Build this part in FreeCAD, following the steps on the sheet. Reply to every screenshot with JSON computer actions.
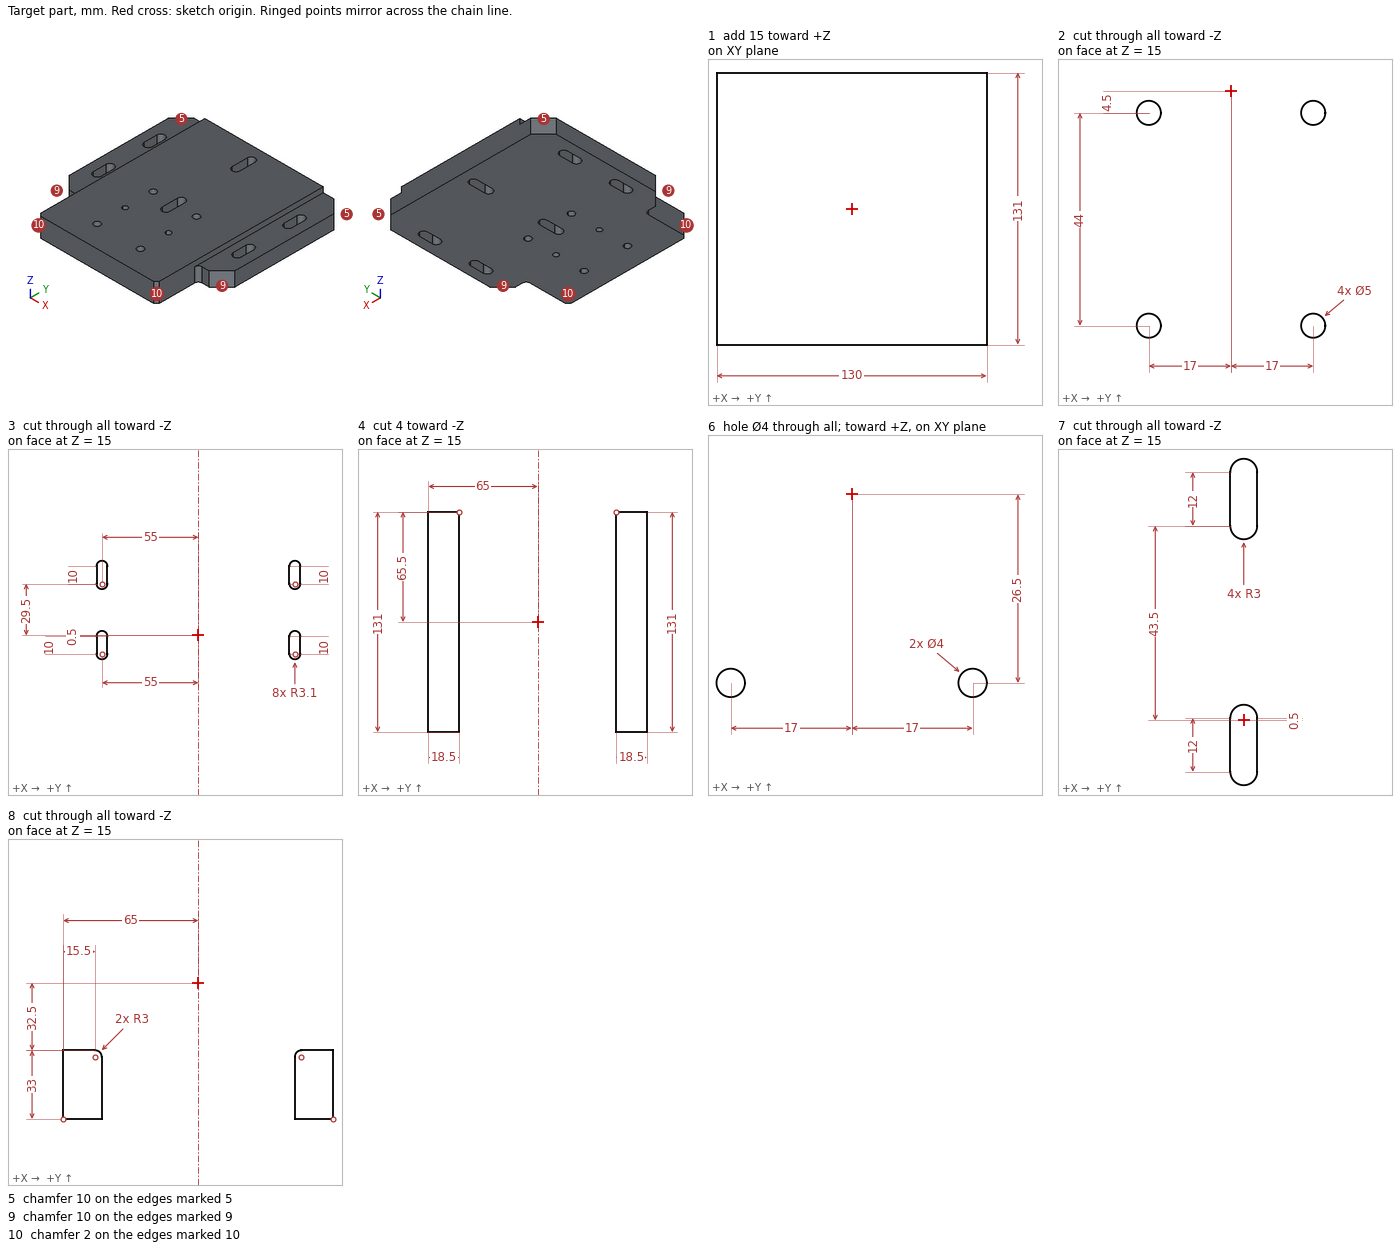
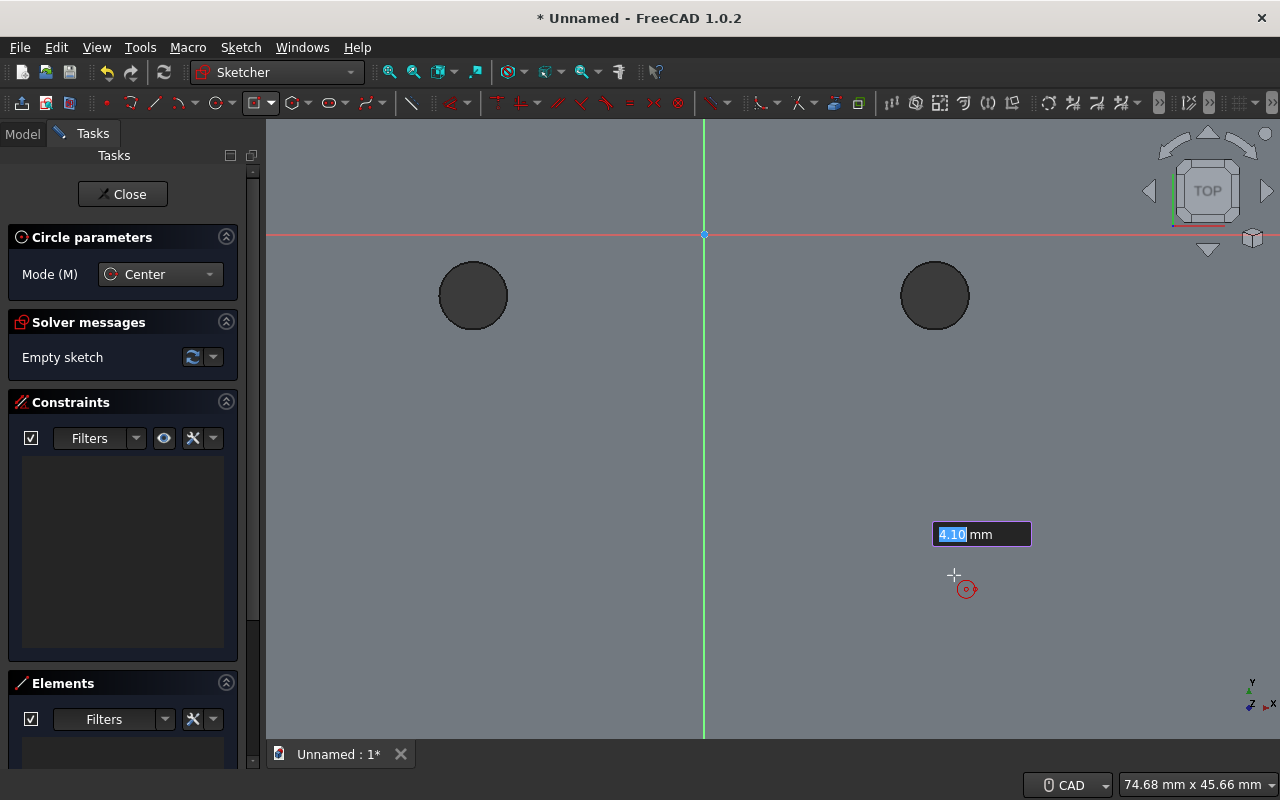
{"action": "type", "text": "4"}
{"action": "key", "text": "Return"}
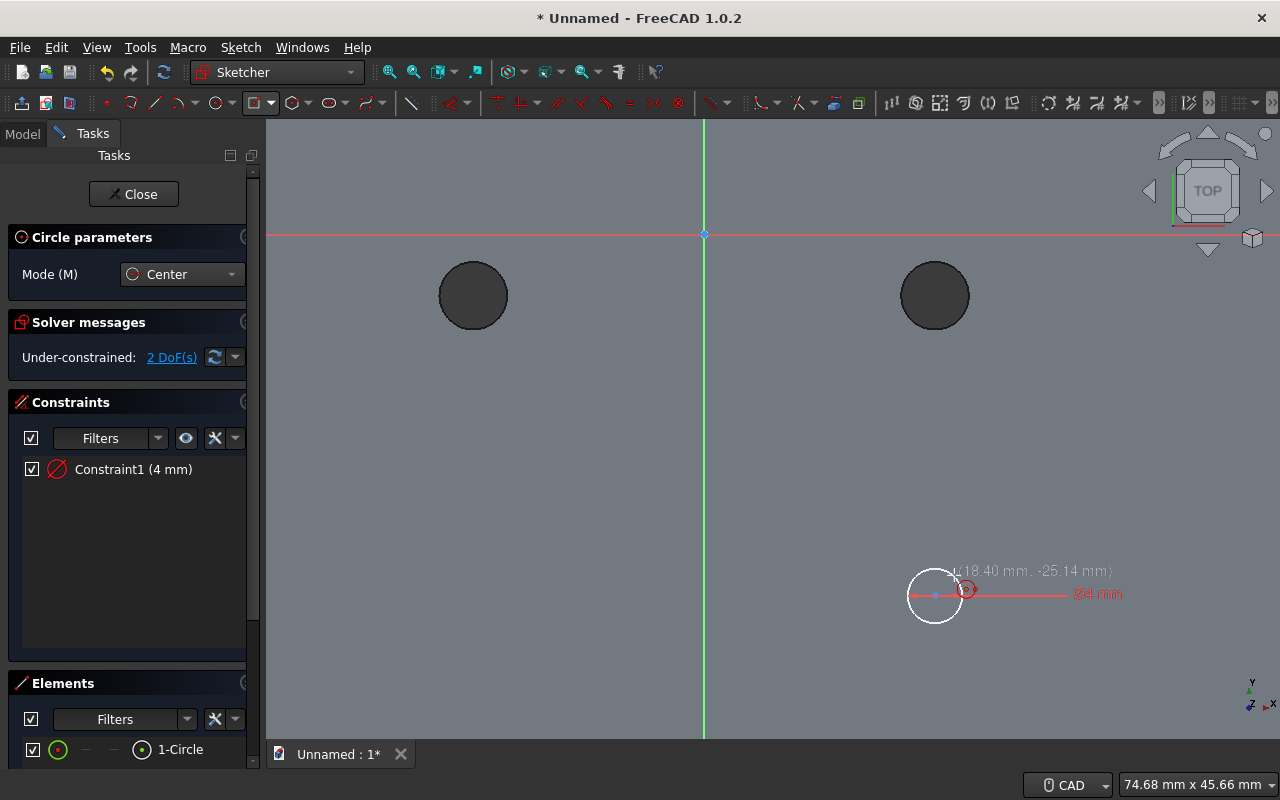
{"action": "left_click", "coordinate": [473, 595]}
{"action": "mouse_move", "coordinate": [493, 575]}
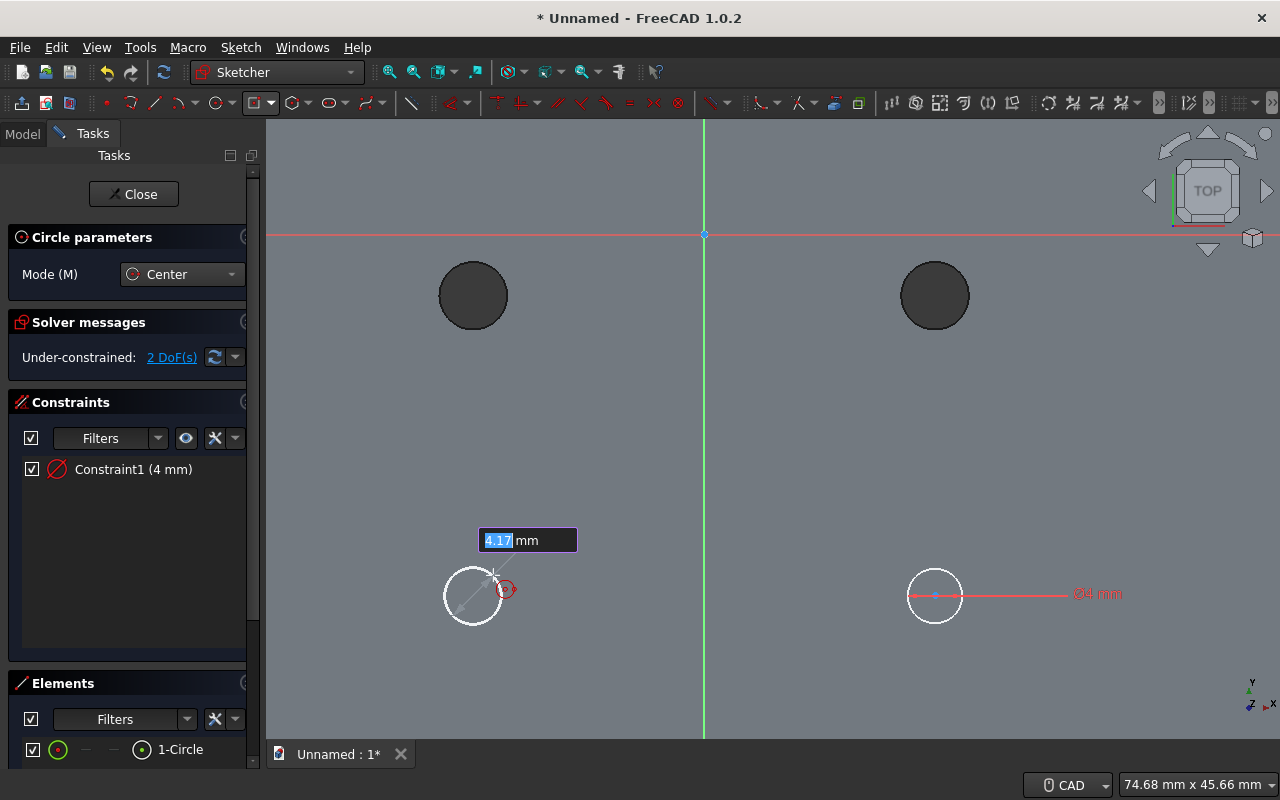
{"action": "type", "text": "4"}
{"action": "key", "text": "Return"}
{"action": "key", "text": "Escape"}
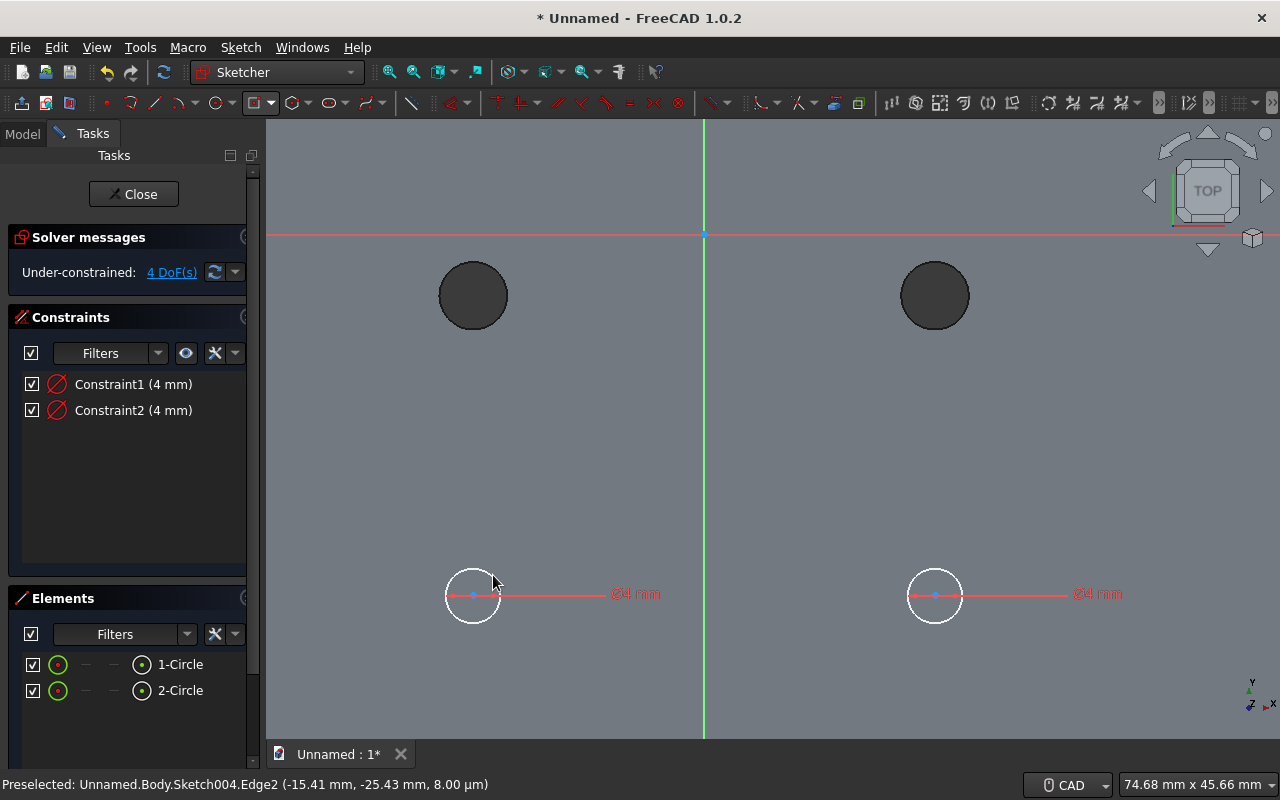
{"action": "left_click", "coordinate": [935, 596]}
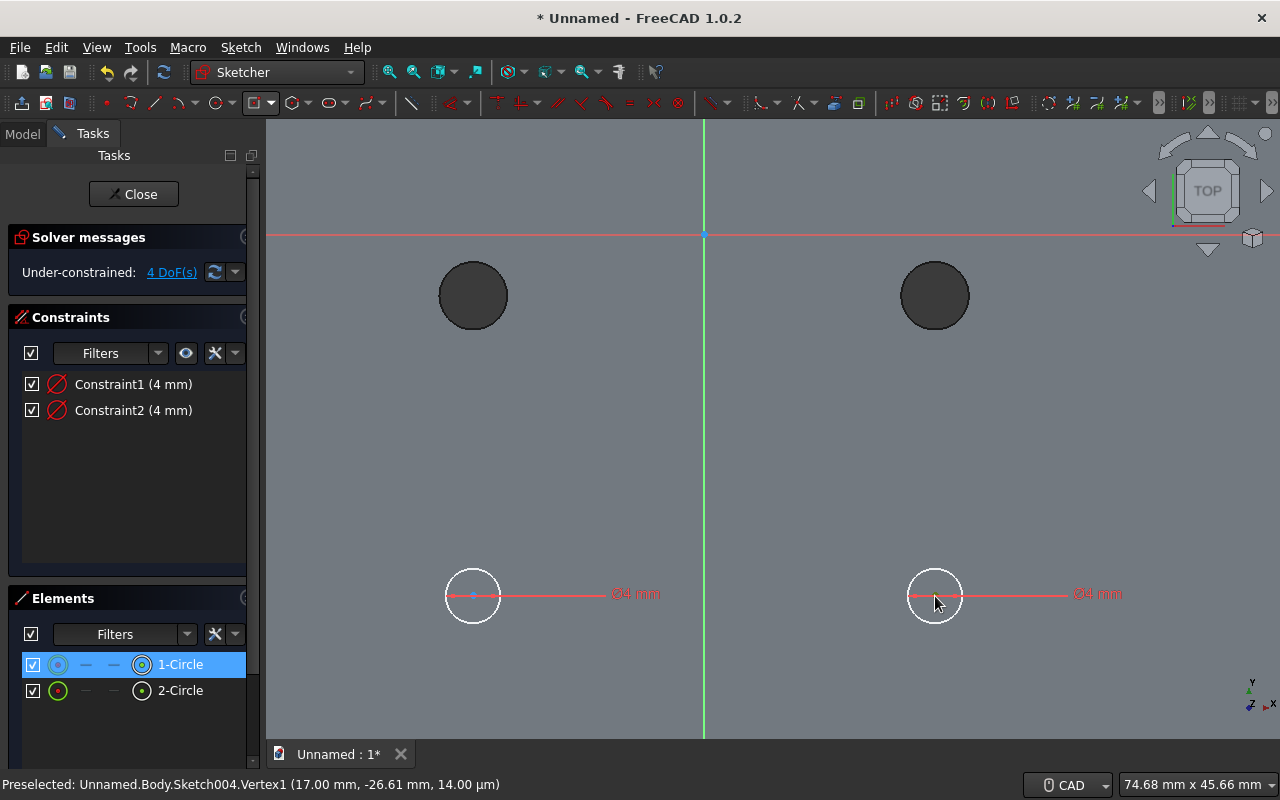
{"action": "left_click", "coordinate": [473, 596]}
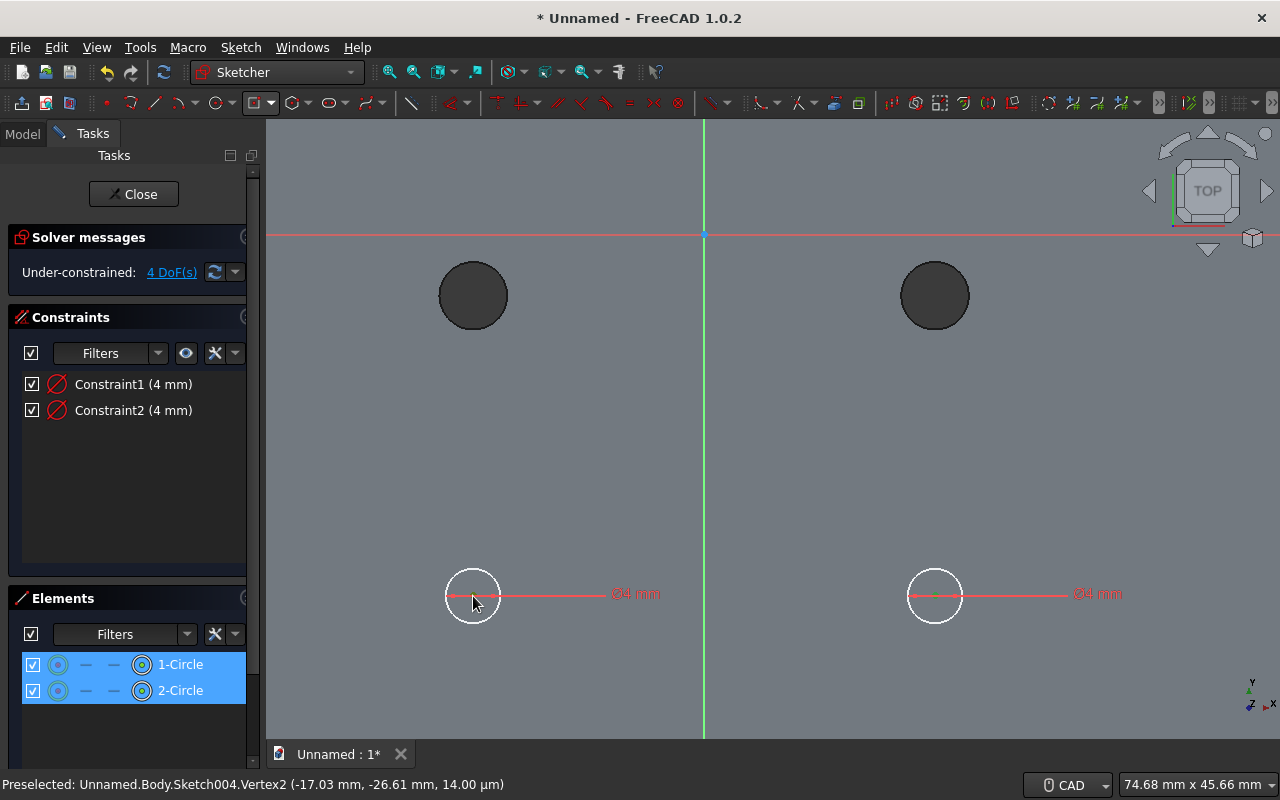
{"action": "key", "text": "h"}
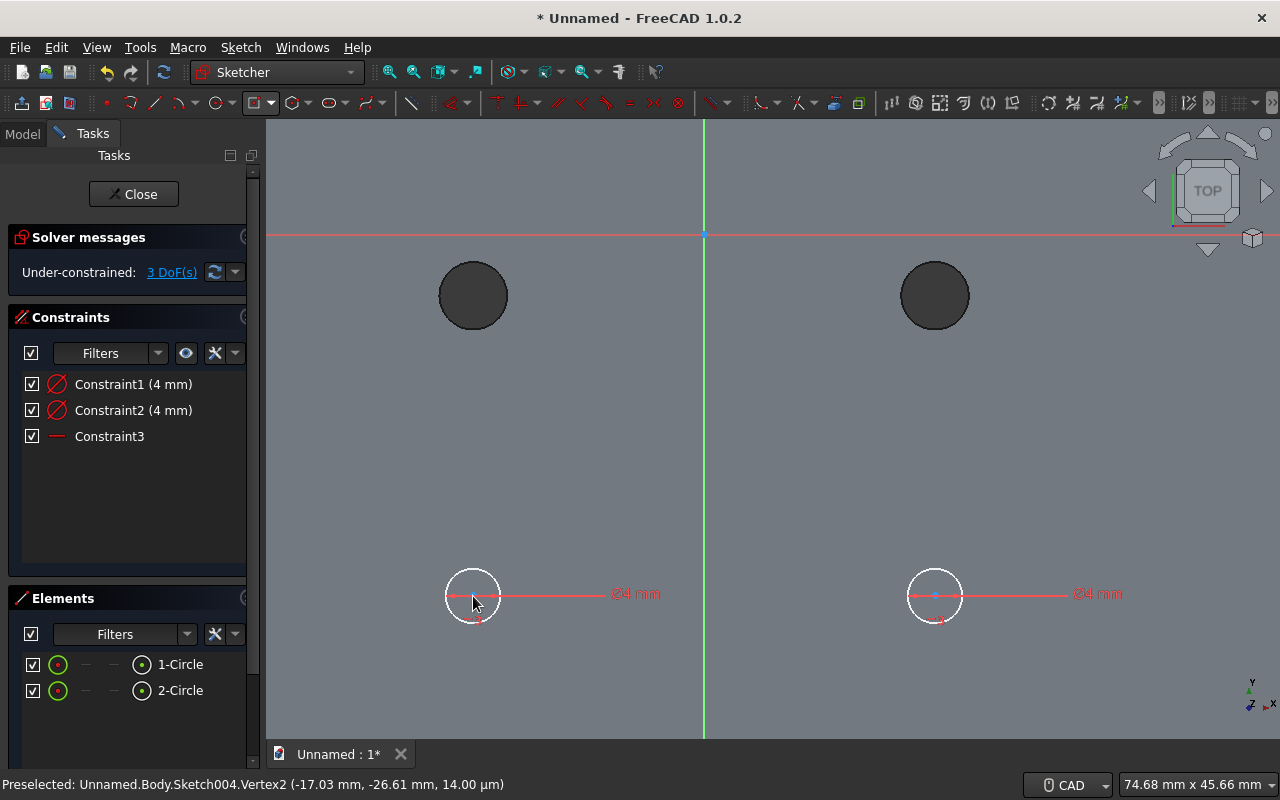
{"action": "left_click", "coordinate": [450, 104]}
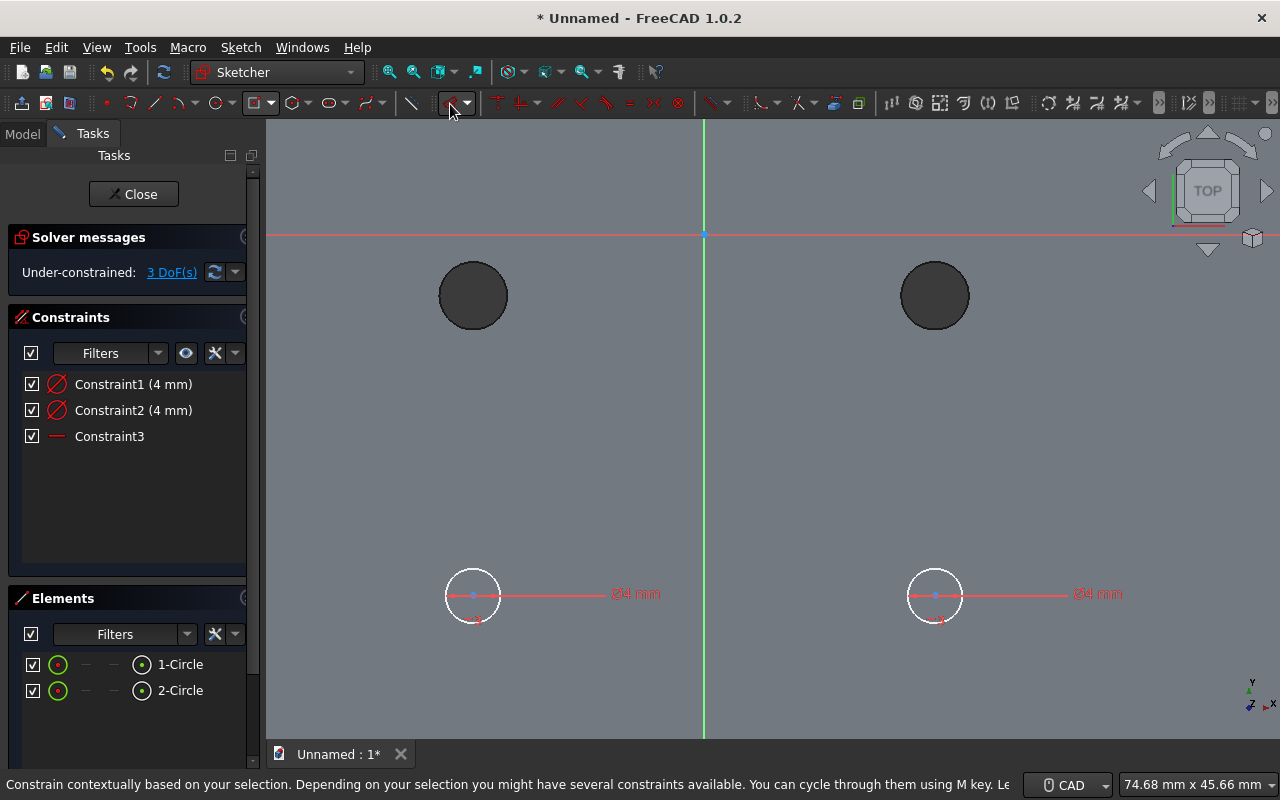
{"action": "left_click", "coordinate": [935, 596]}
{"action": "left_click", "coordinate": [820, 201]}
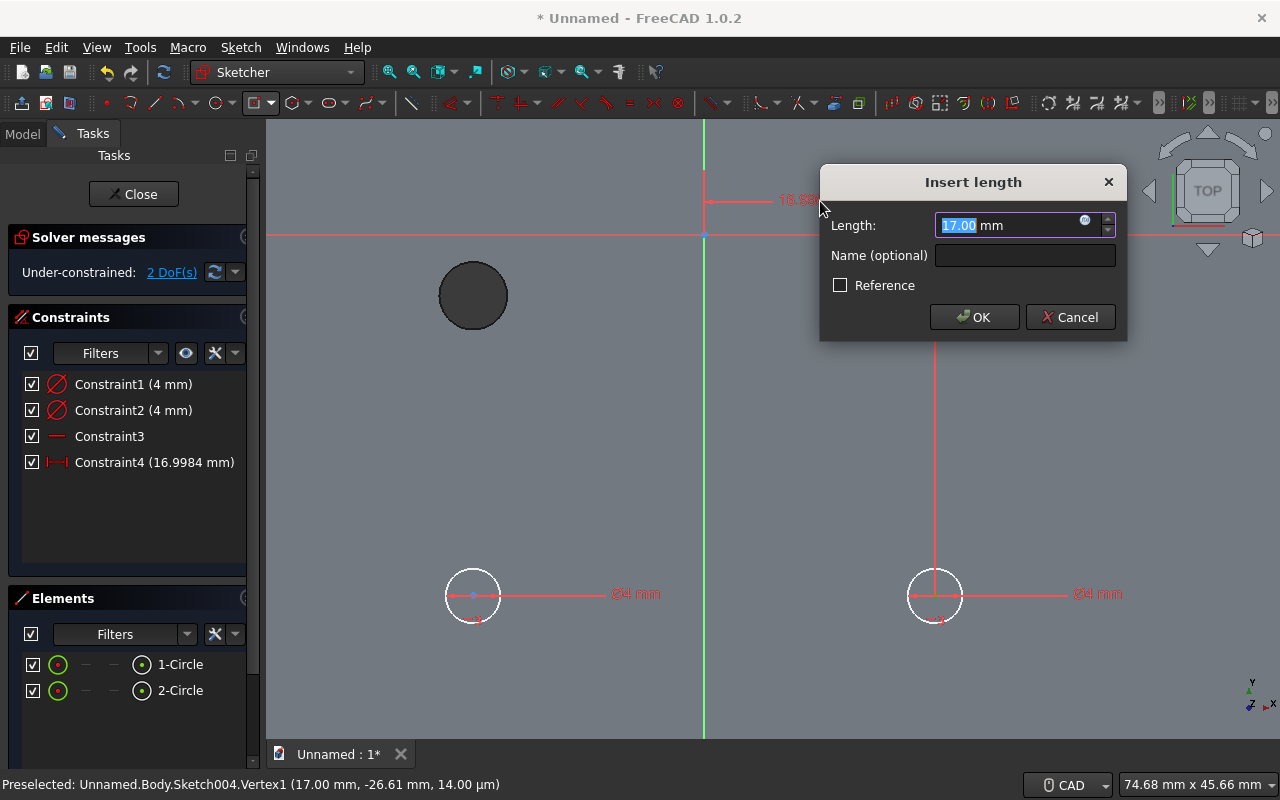
{"action": "type", "text": "17"}
{"action": "key", "text": "Return"}